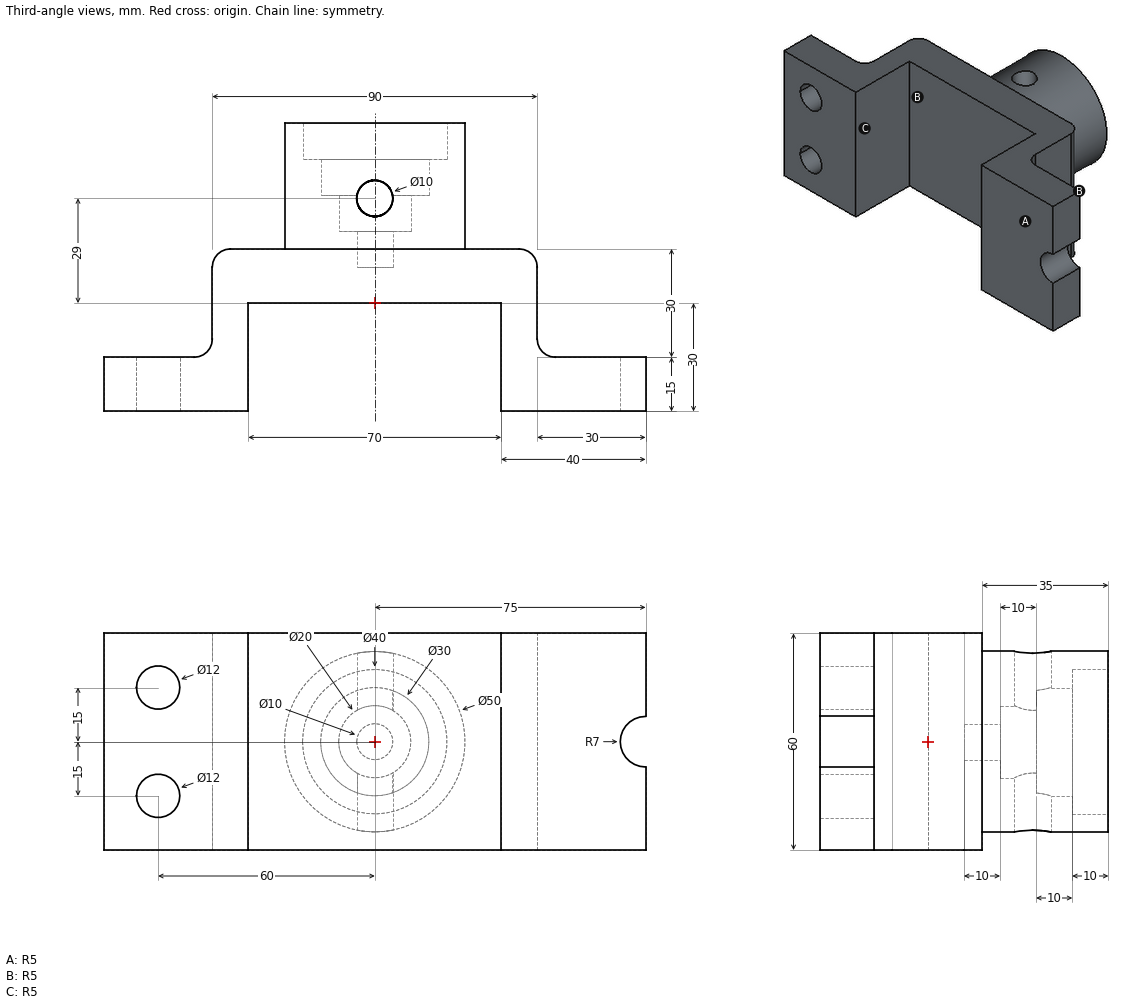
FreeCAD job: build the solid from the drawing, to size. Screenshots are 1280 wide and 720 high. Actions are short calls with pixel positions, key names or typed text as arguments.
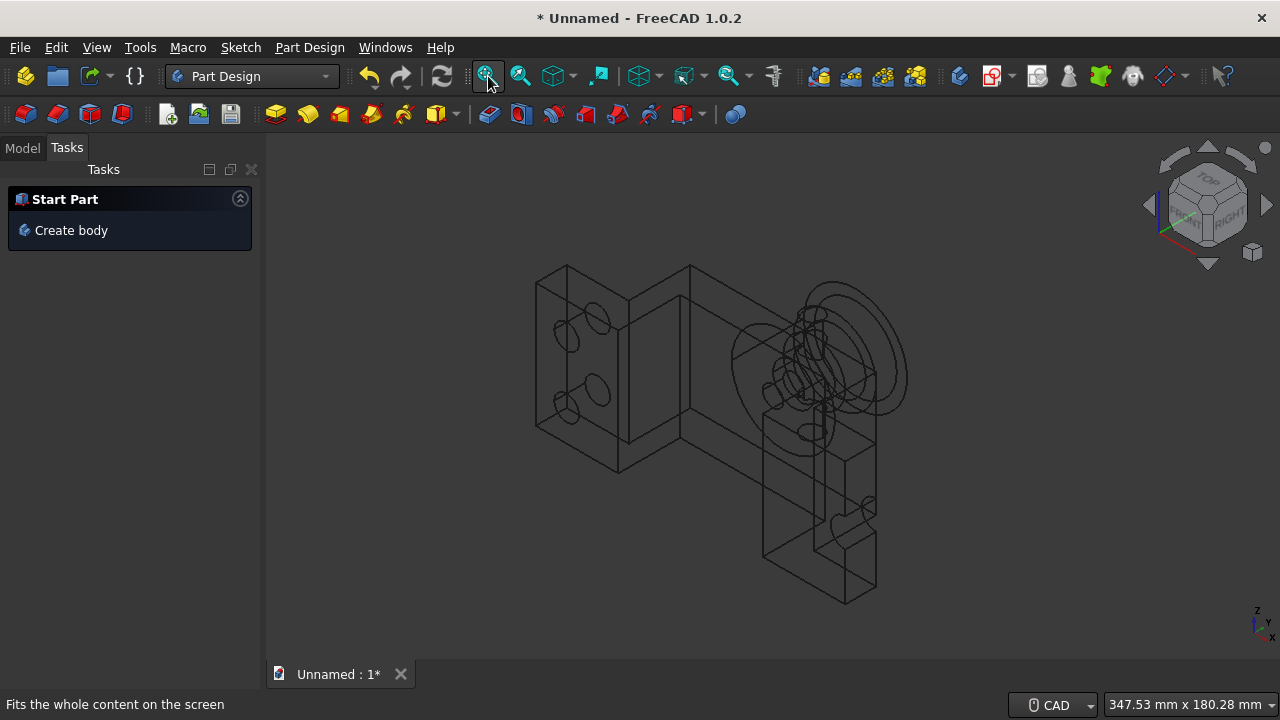
click(814, 478)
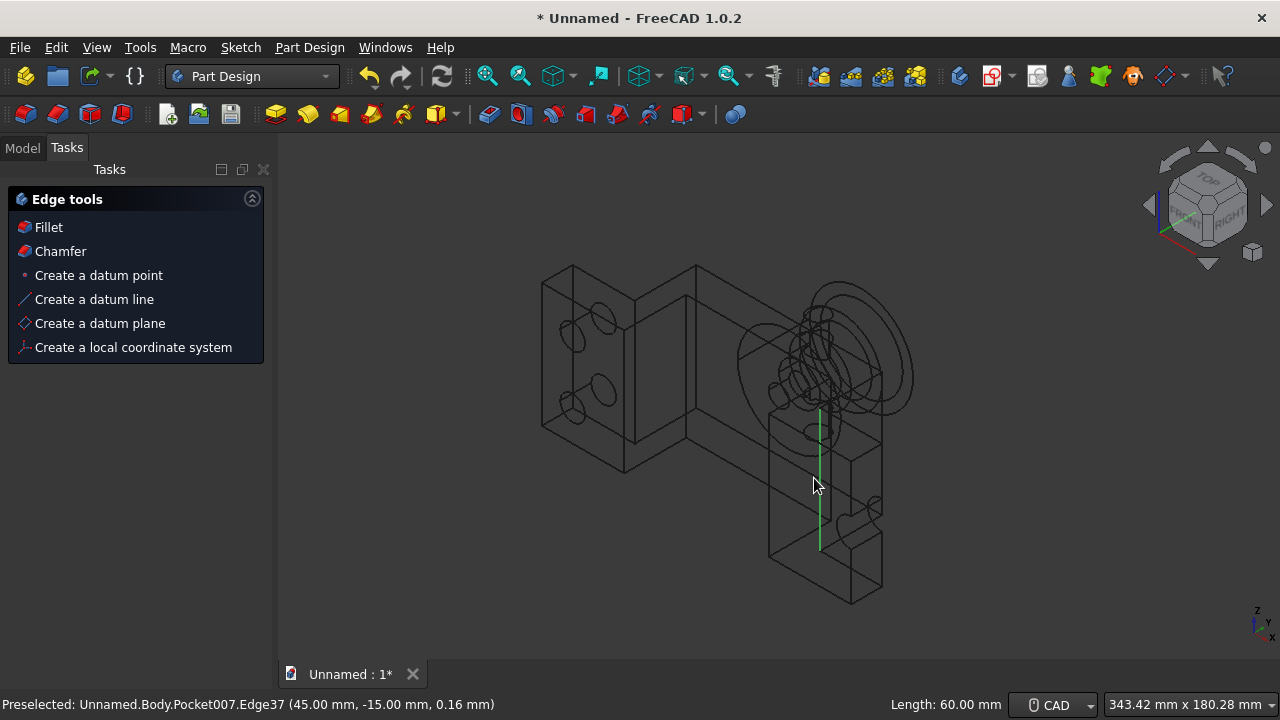
key(v)
key(1)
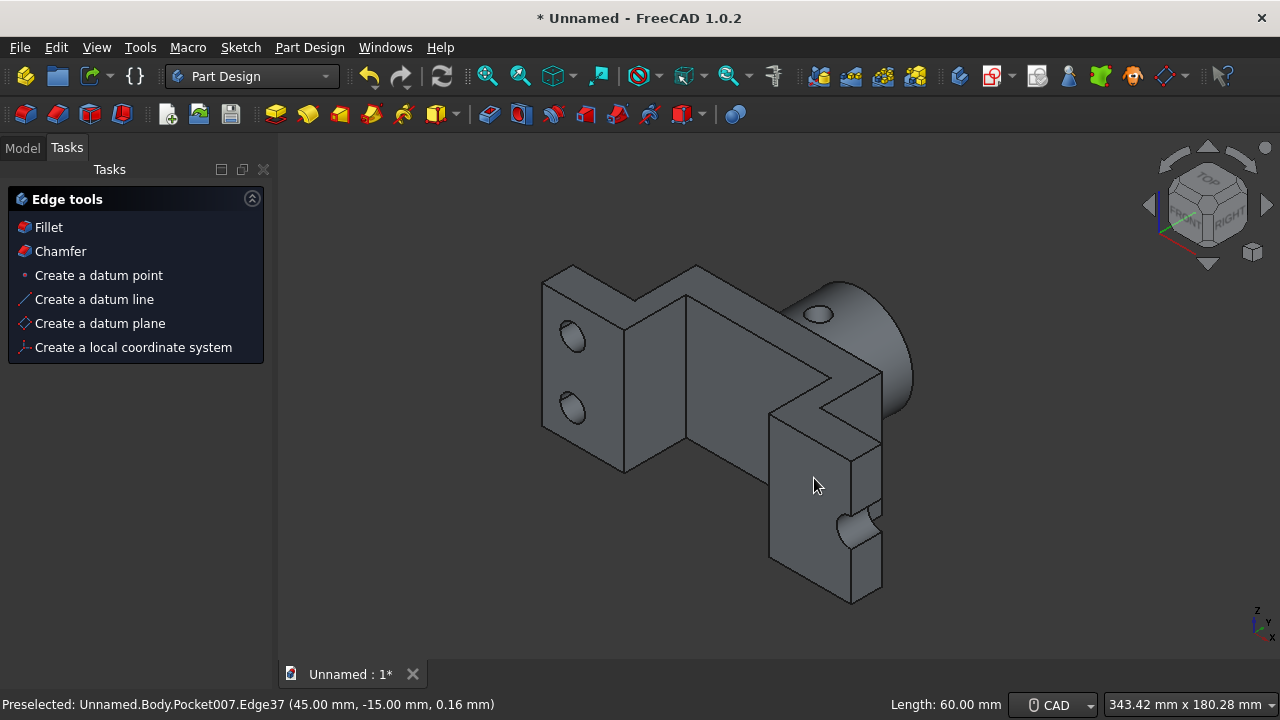
click(26, 114)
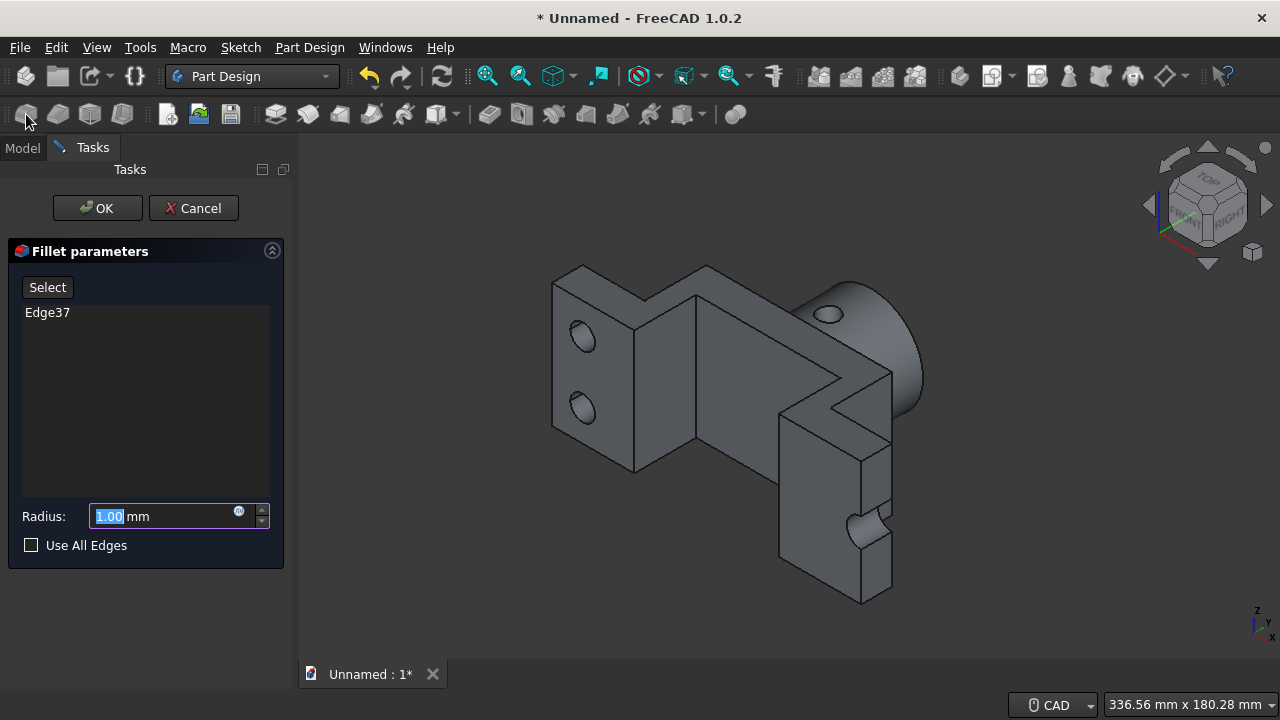
text(5)
key(Tab)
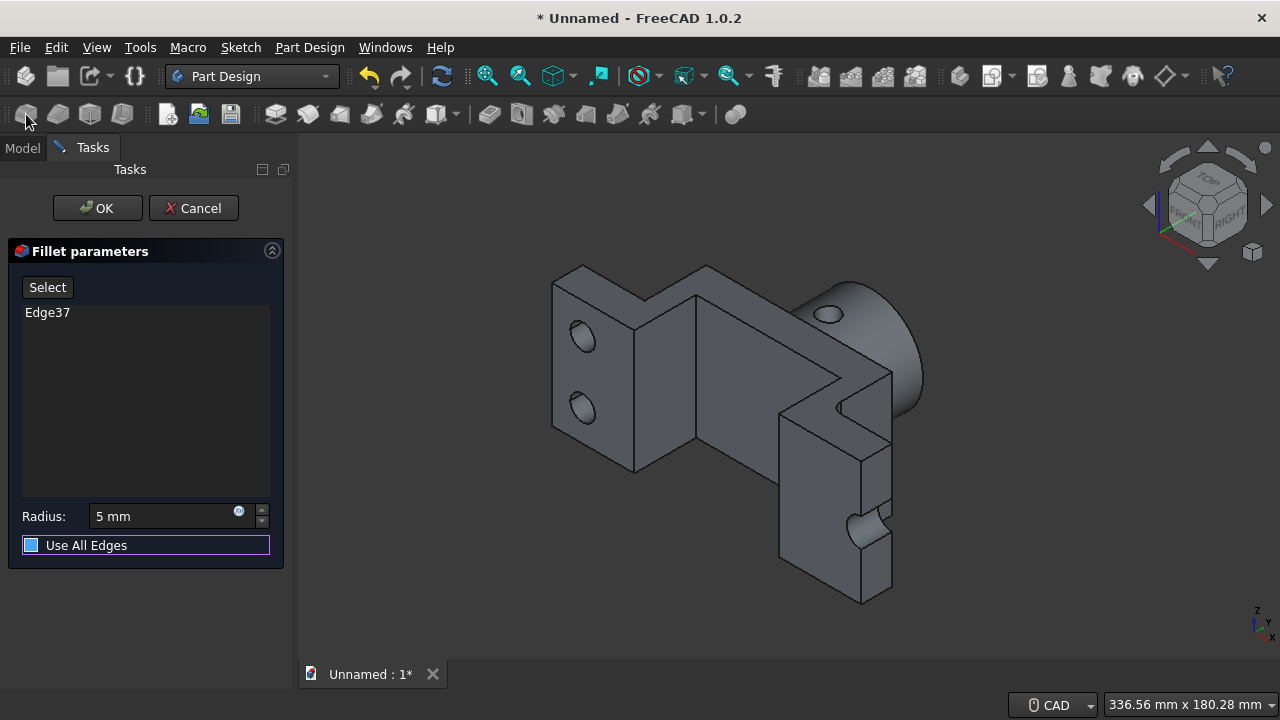
click(98, 208)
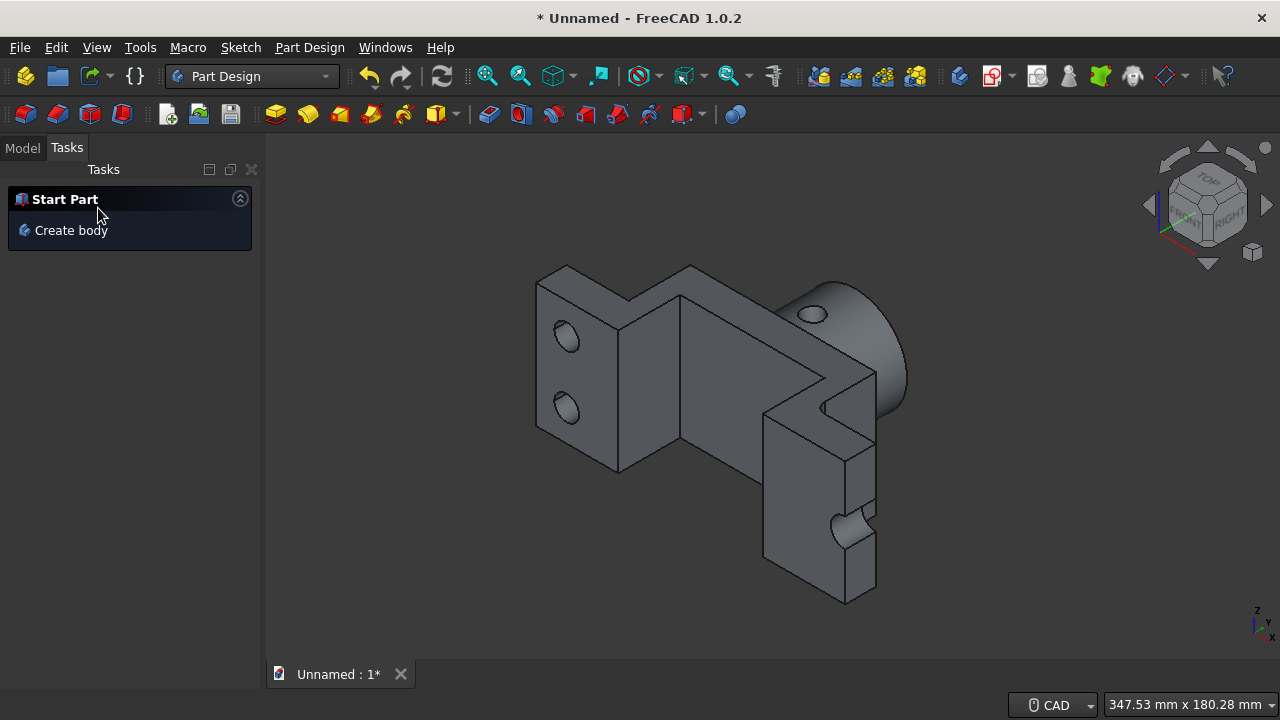
key(2)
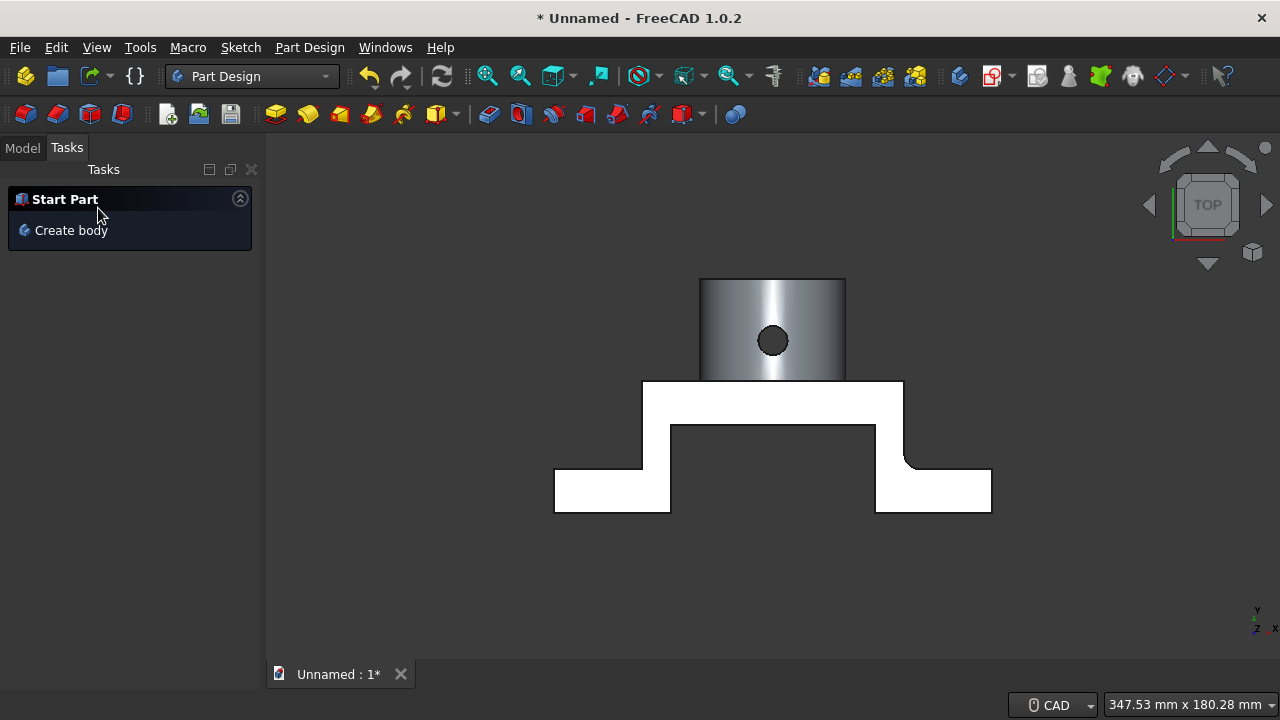
click(488, 76)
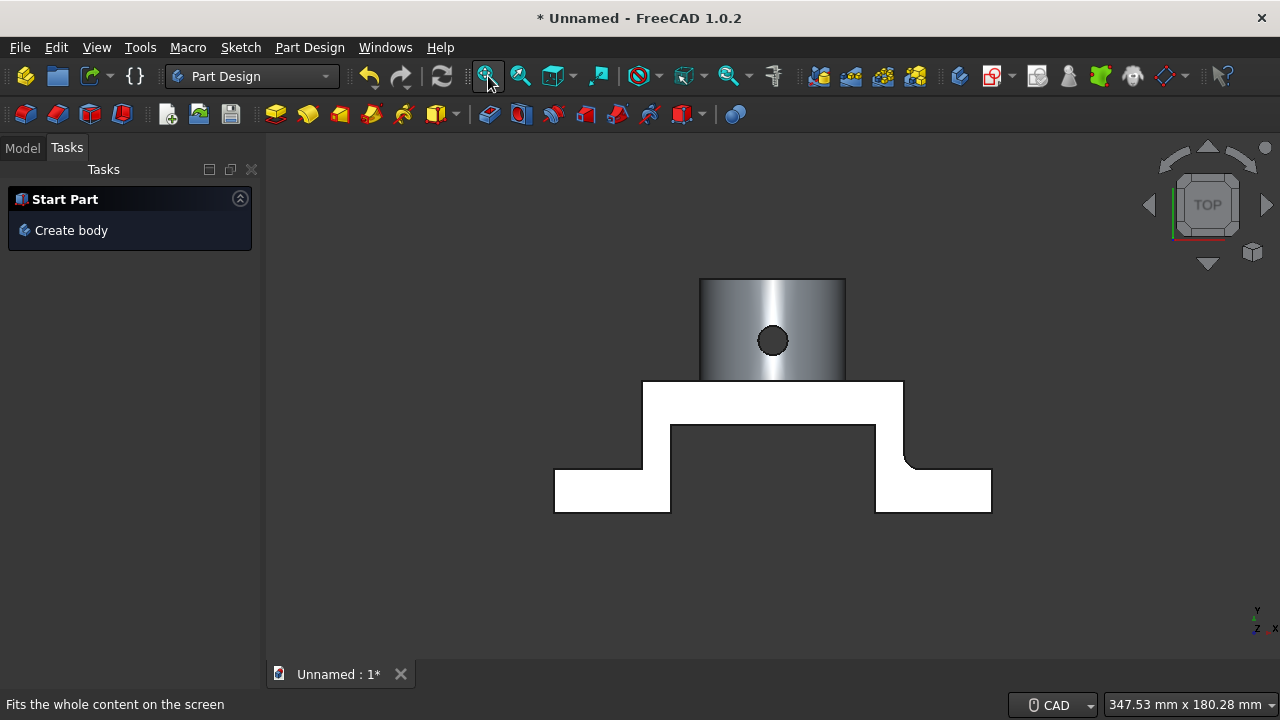
key(0)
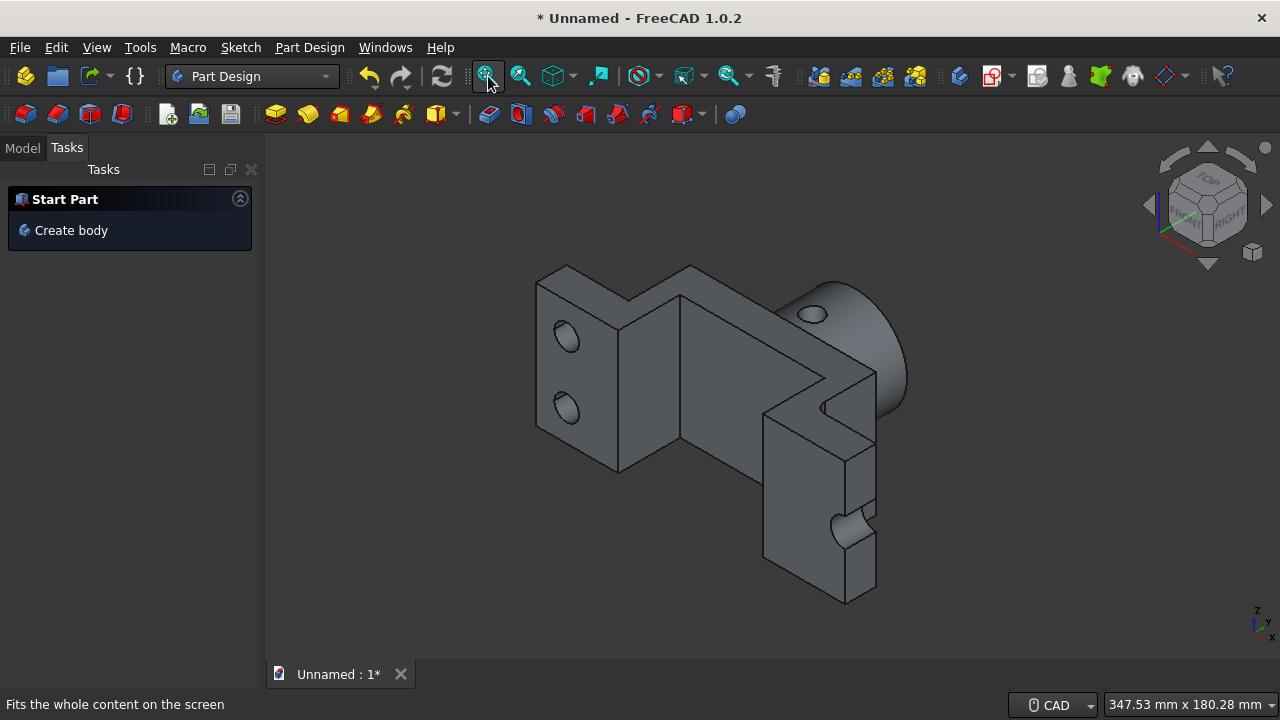
key(1)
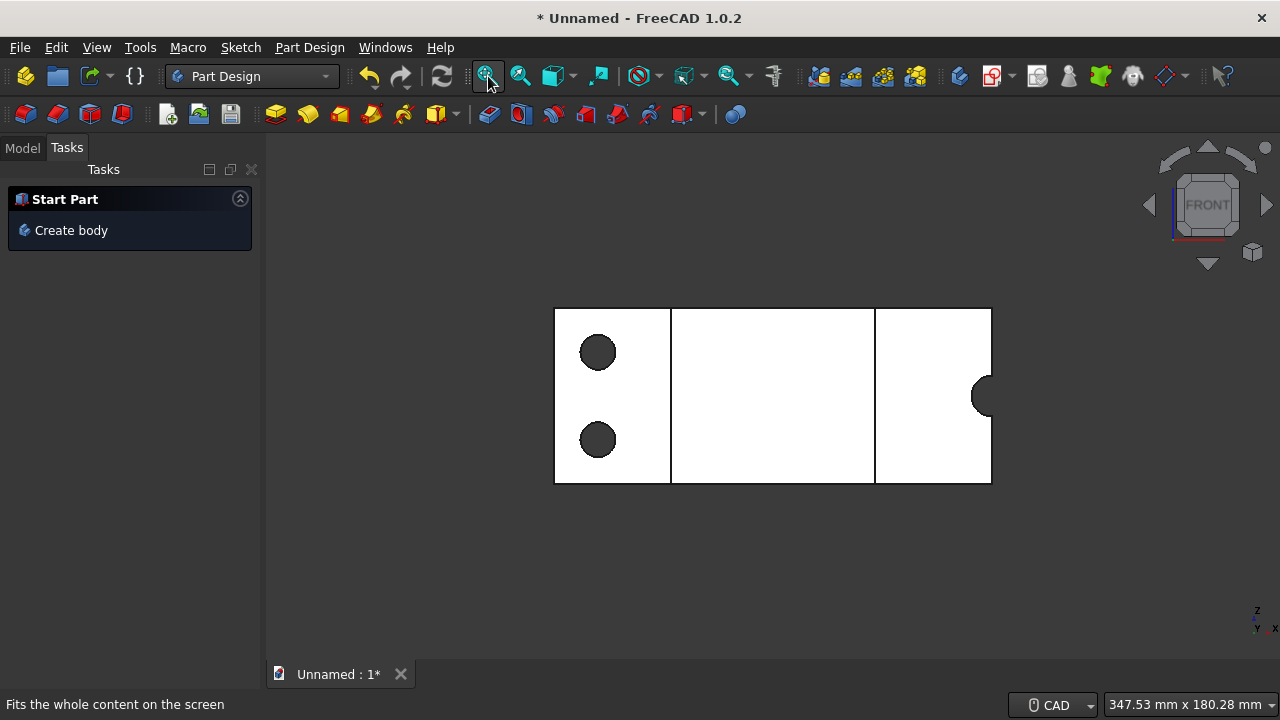
click(488, 76)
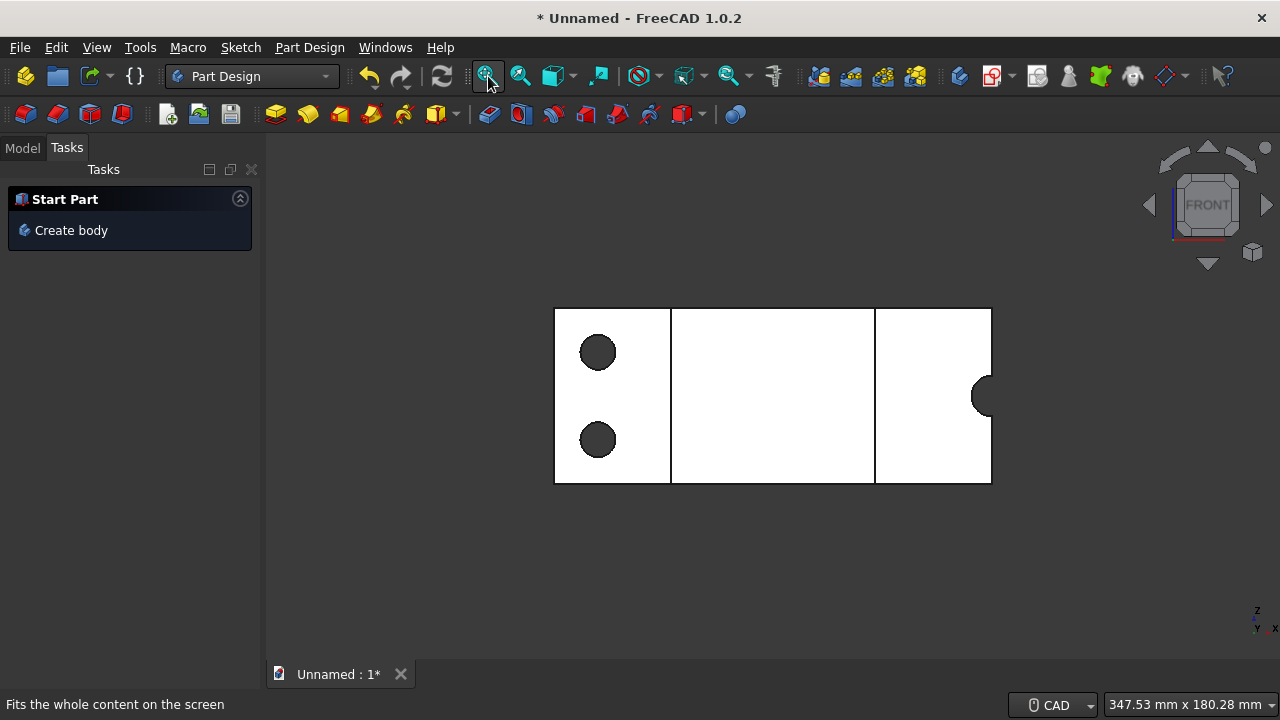
key(3)